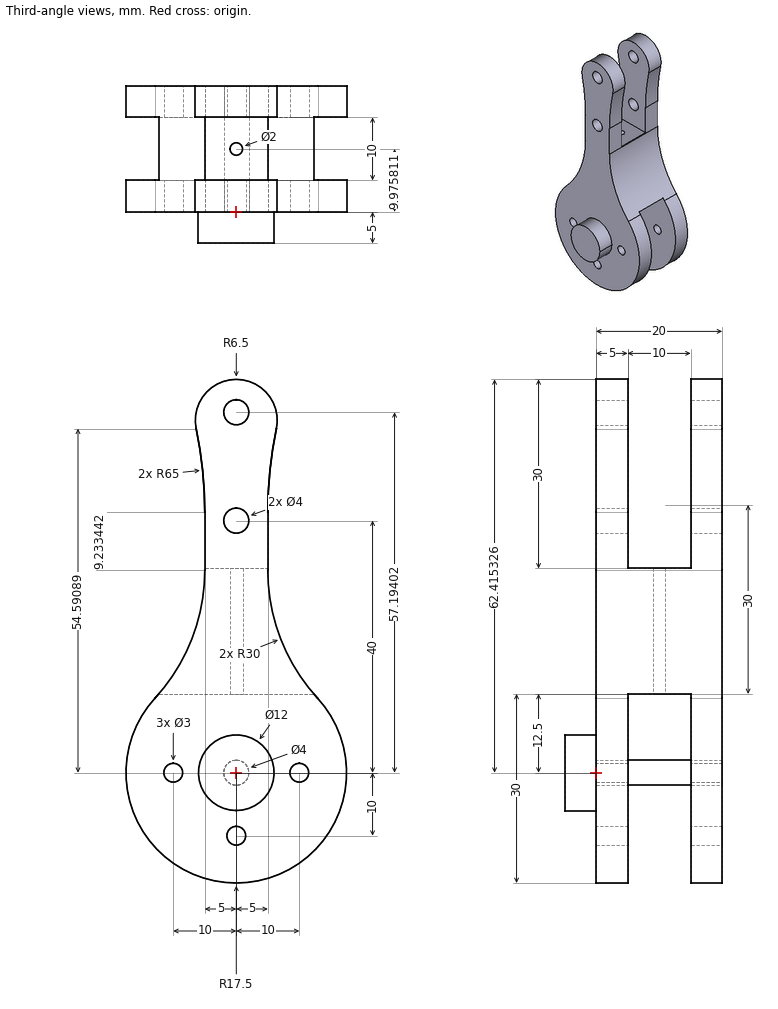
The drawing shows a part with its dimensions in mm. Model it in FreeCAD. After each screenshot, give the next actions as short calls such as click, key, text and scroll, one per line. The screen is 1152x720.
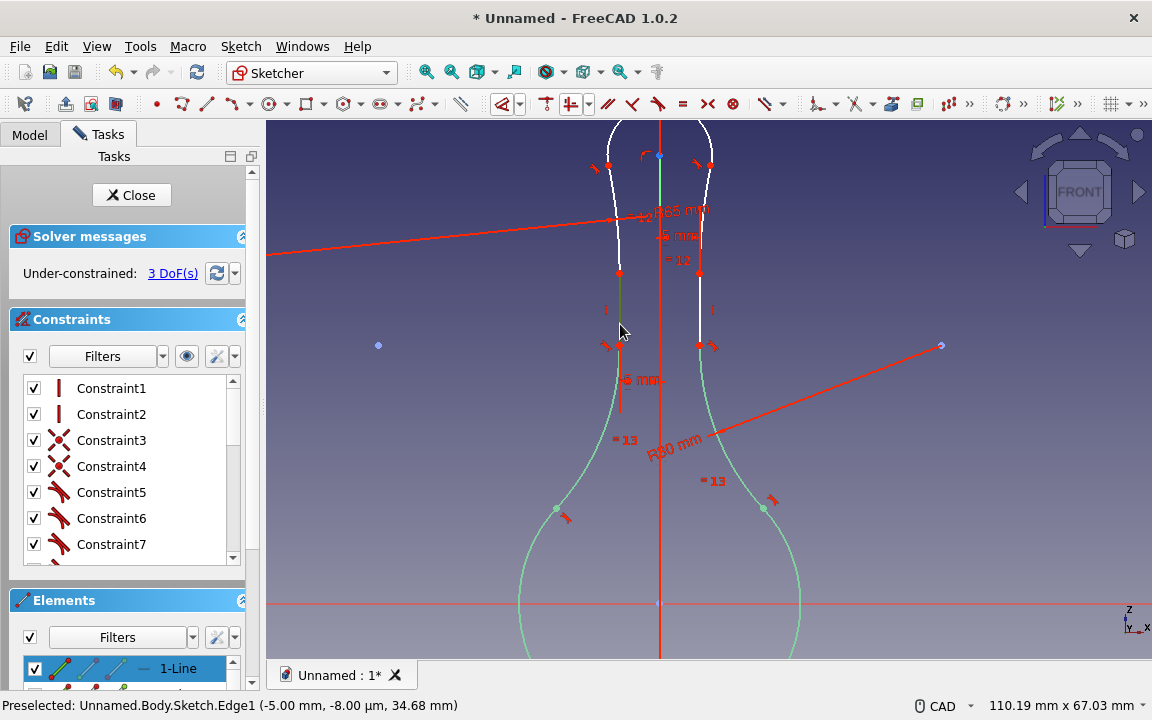
click(520, 104)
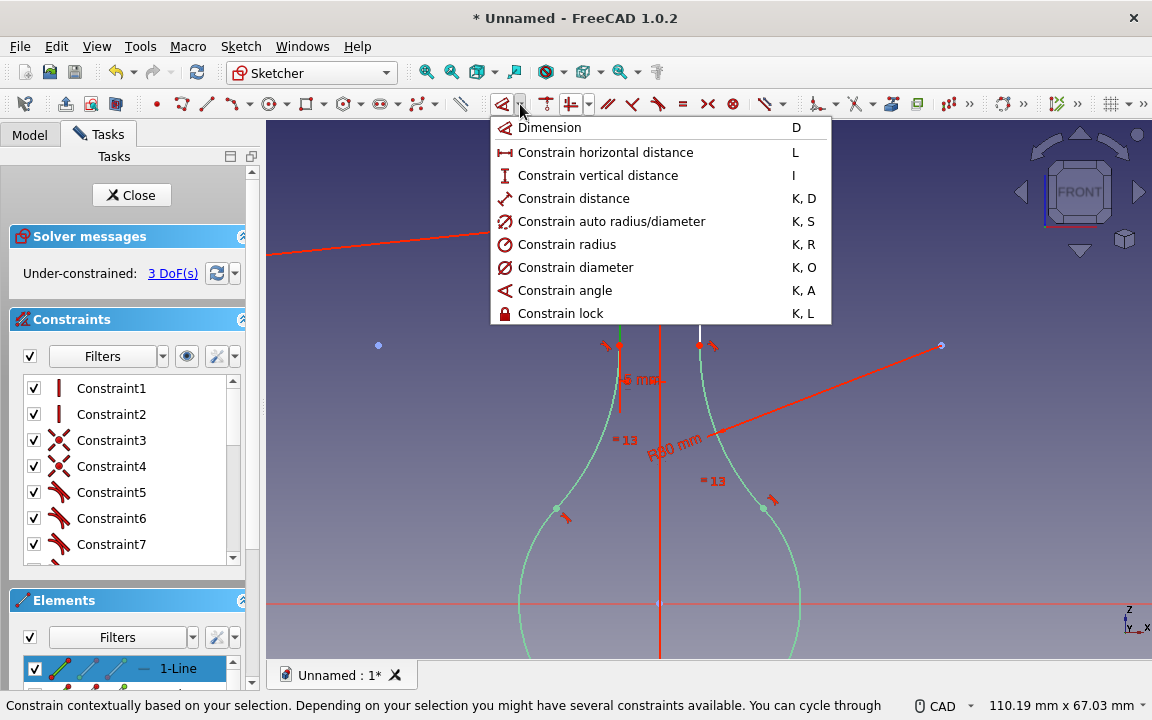
click(661, 176)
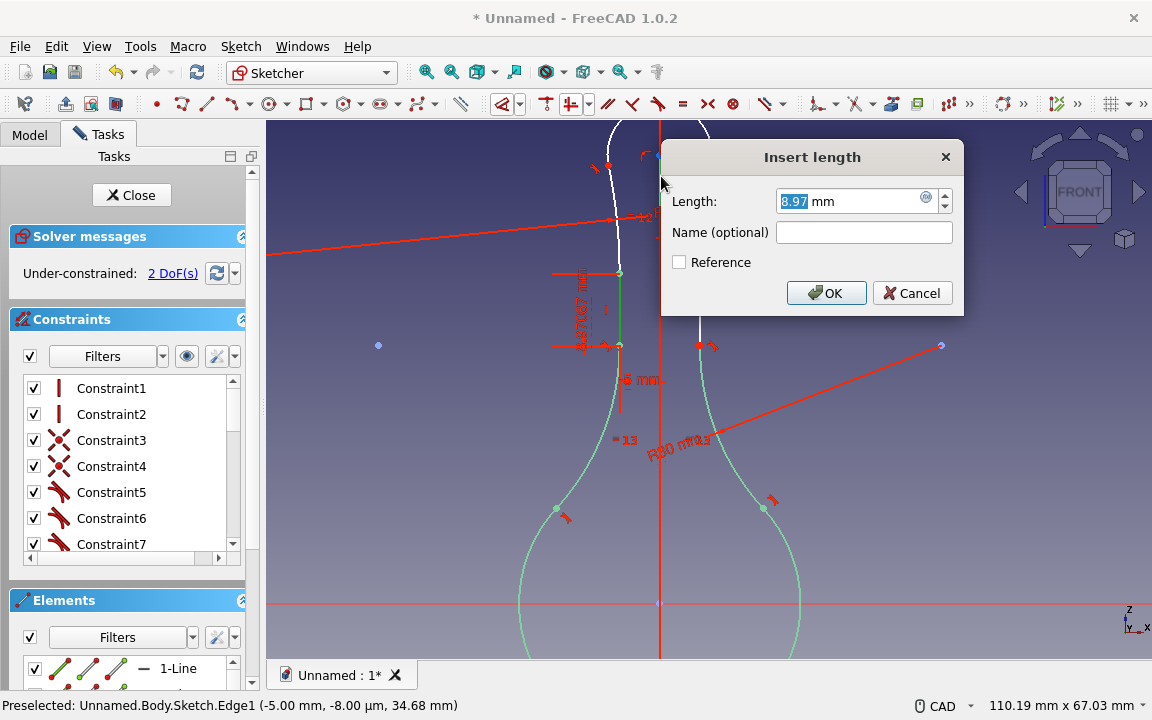
text(9.233442)
key(Return)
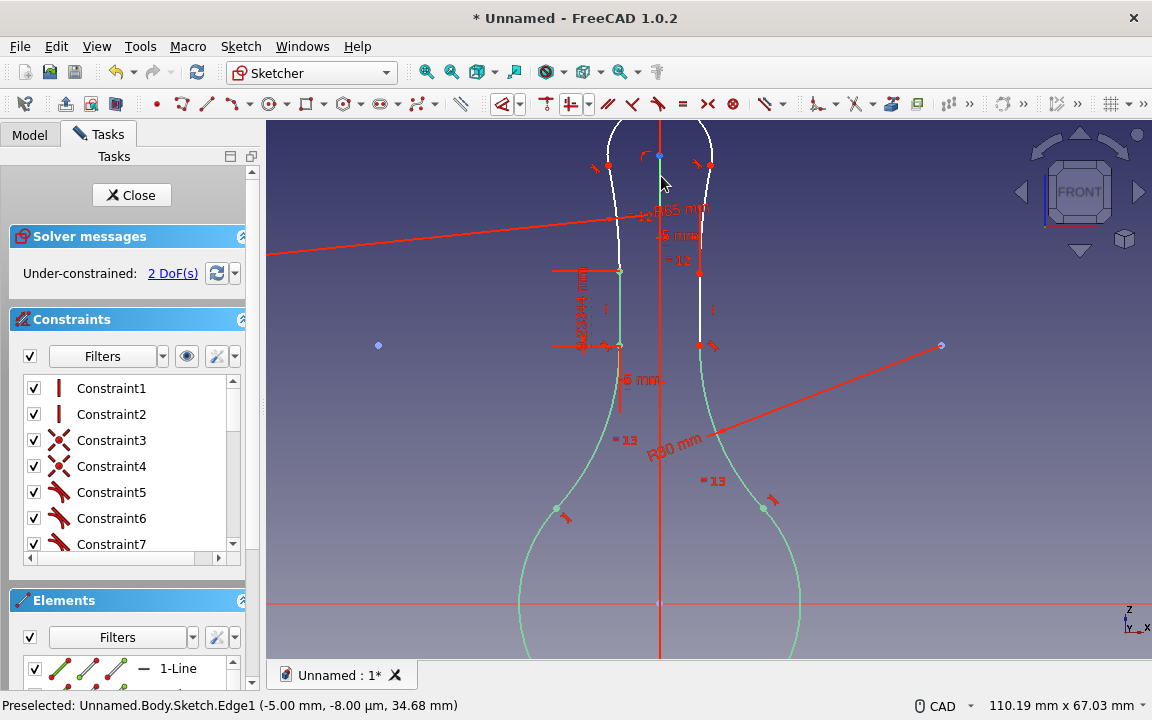
click(700, 295)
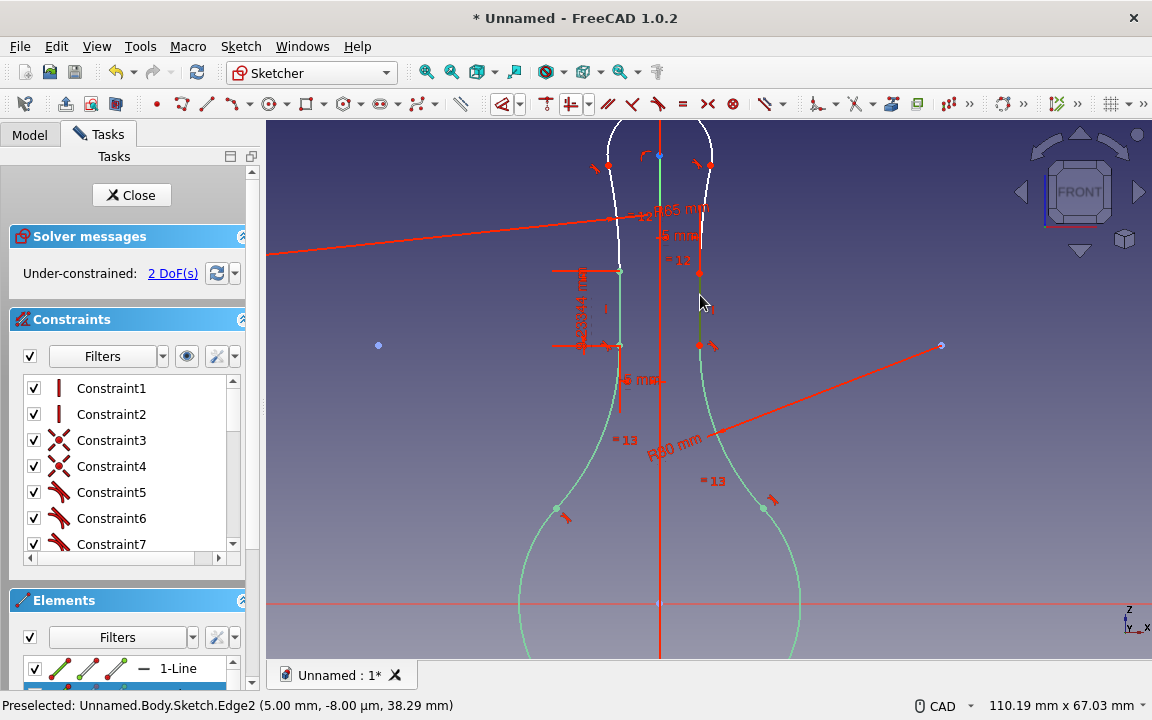
key(i)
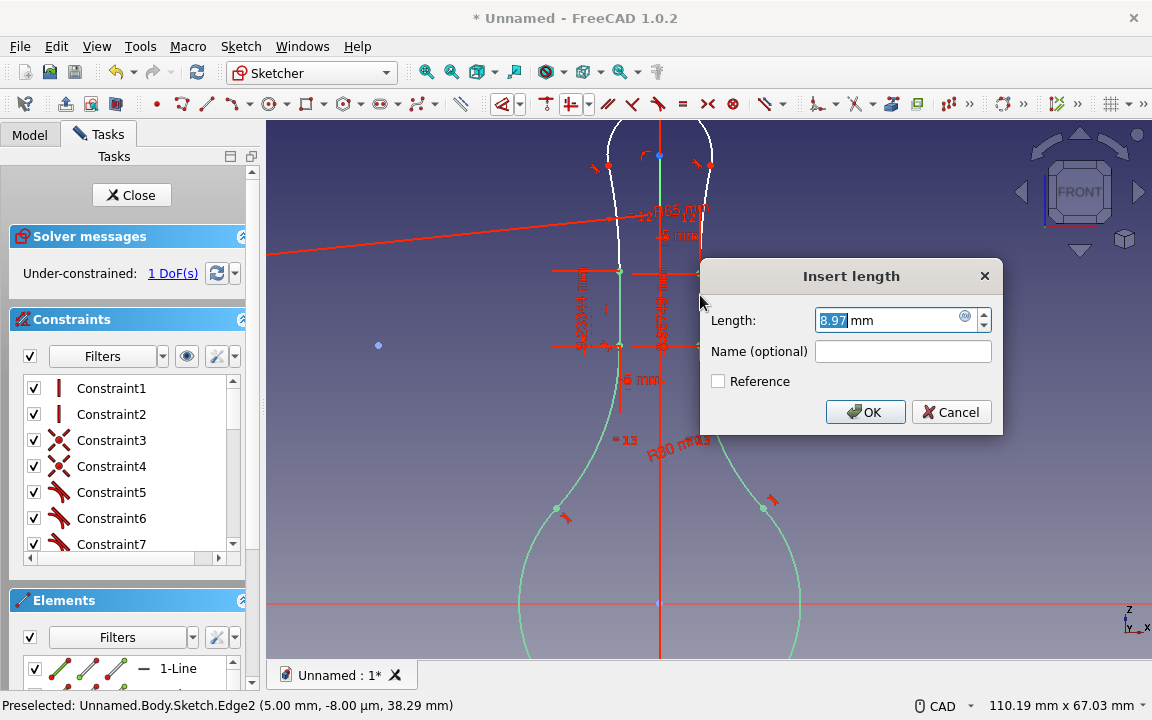
text(9.233442)
key(Return)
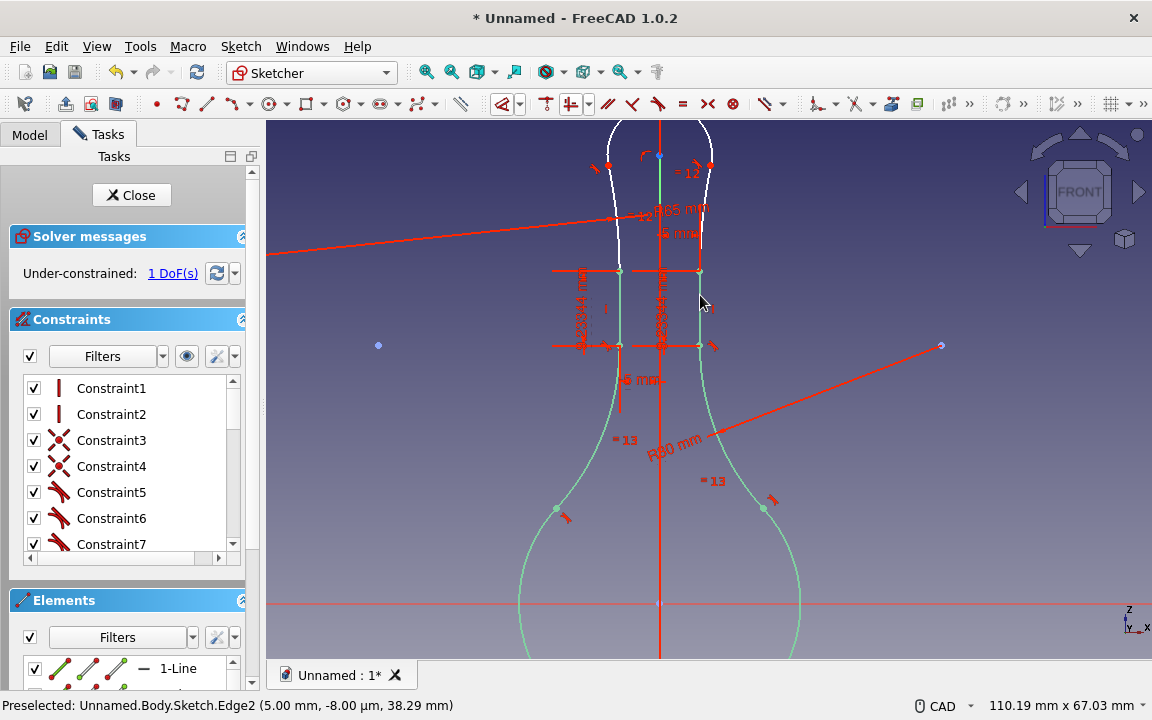
click(609, 166)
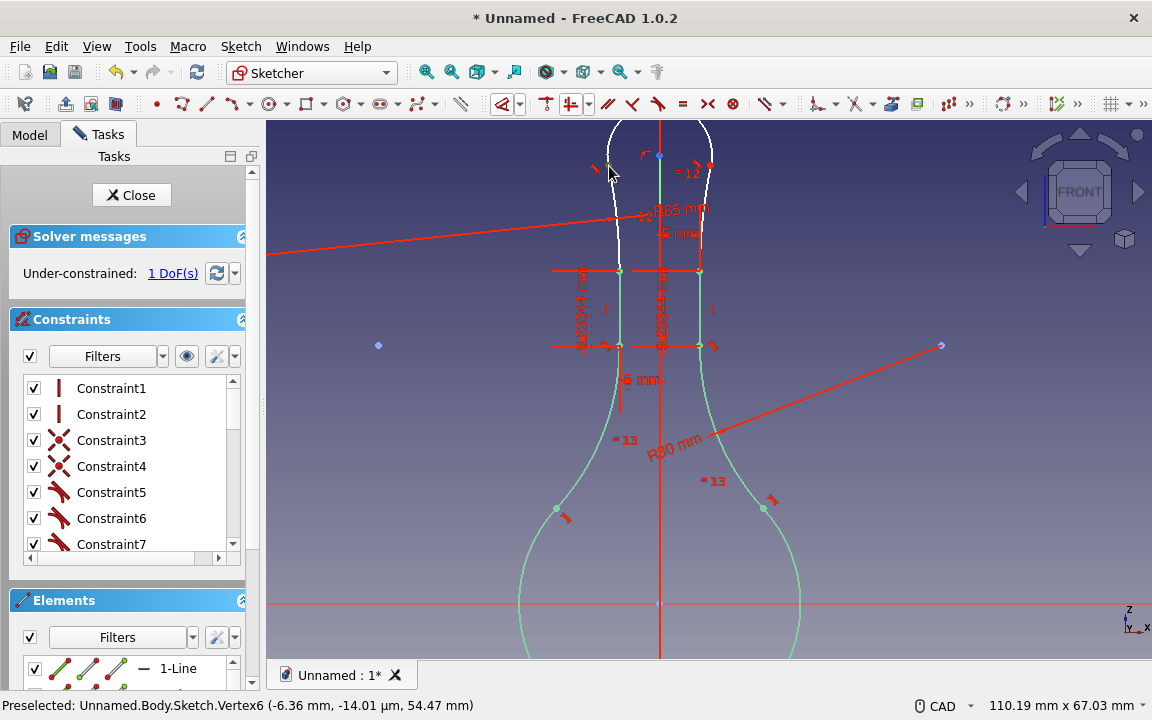
key(i)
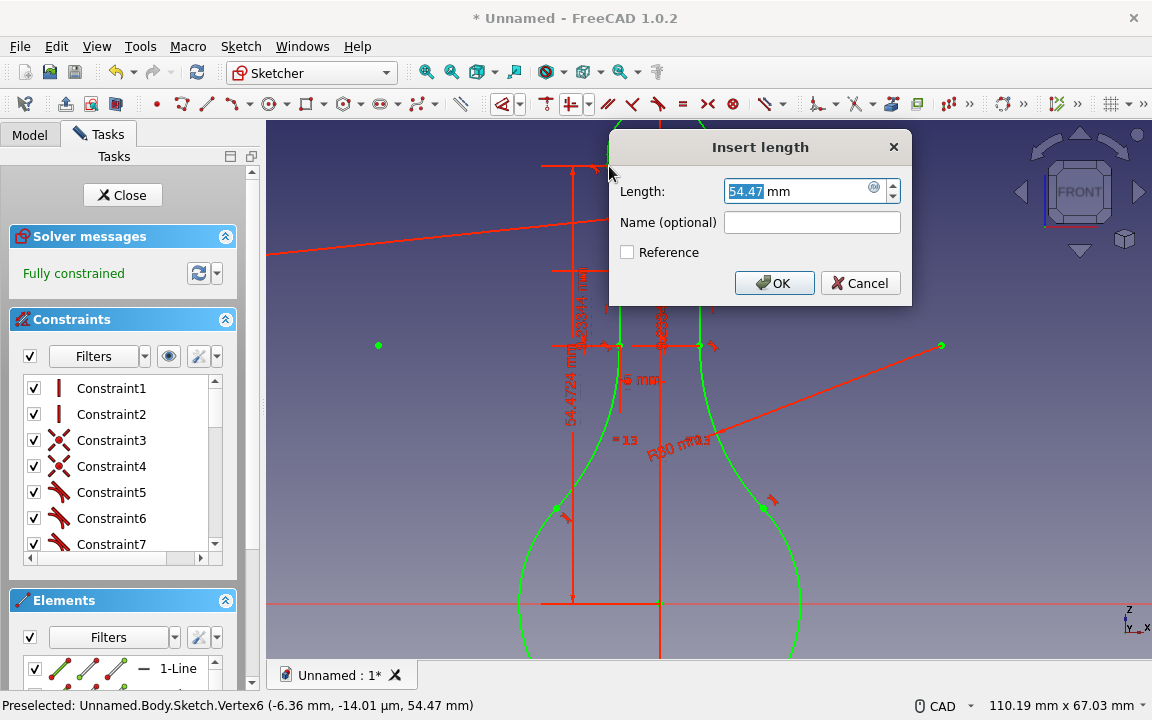
text(54.59089)
key(Return)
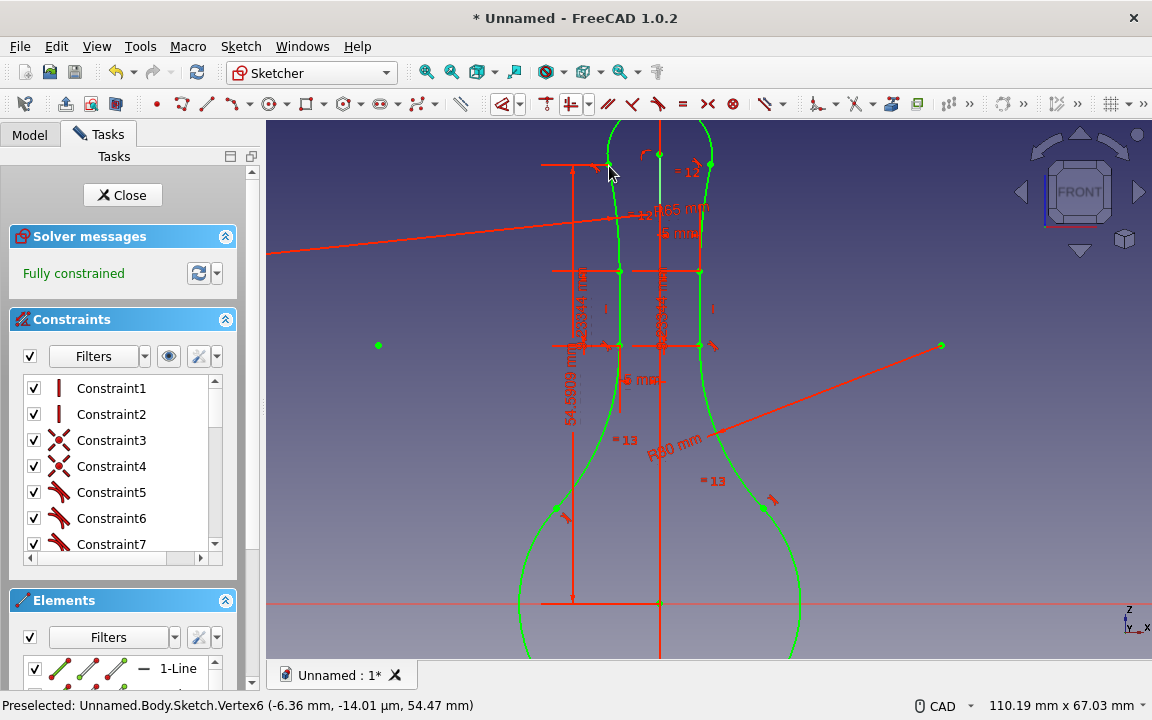
click(123, 195)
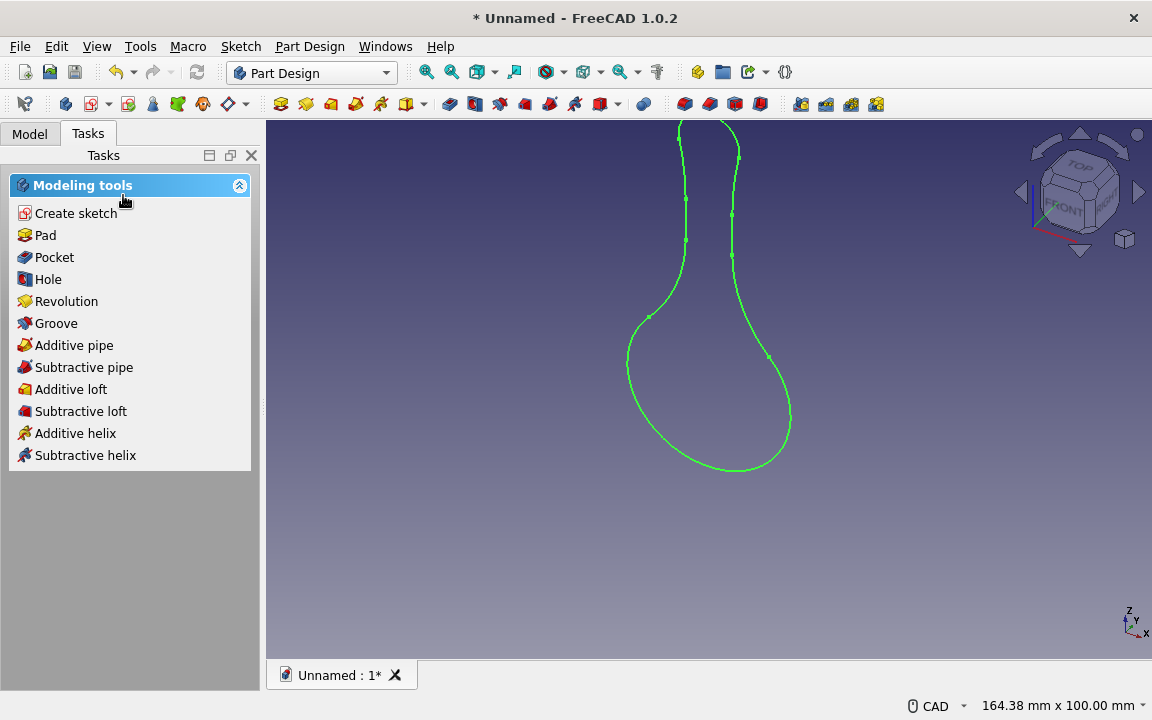
click(281, 104)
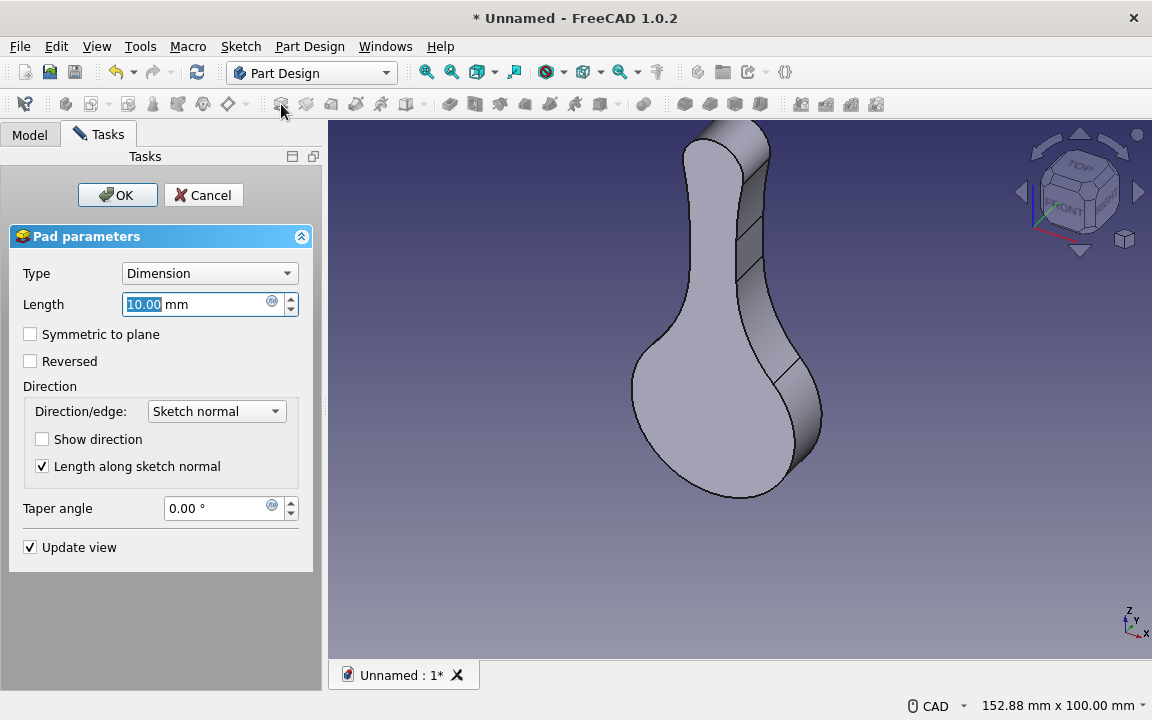
text(20)
key(Tab)